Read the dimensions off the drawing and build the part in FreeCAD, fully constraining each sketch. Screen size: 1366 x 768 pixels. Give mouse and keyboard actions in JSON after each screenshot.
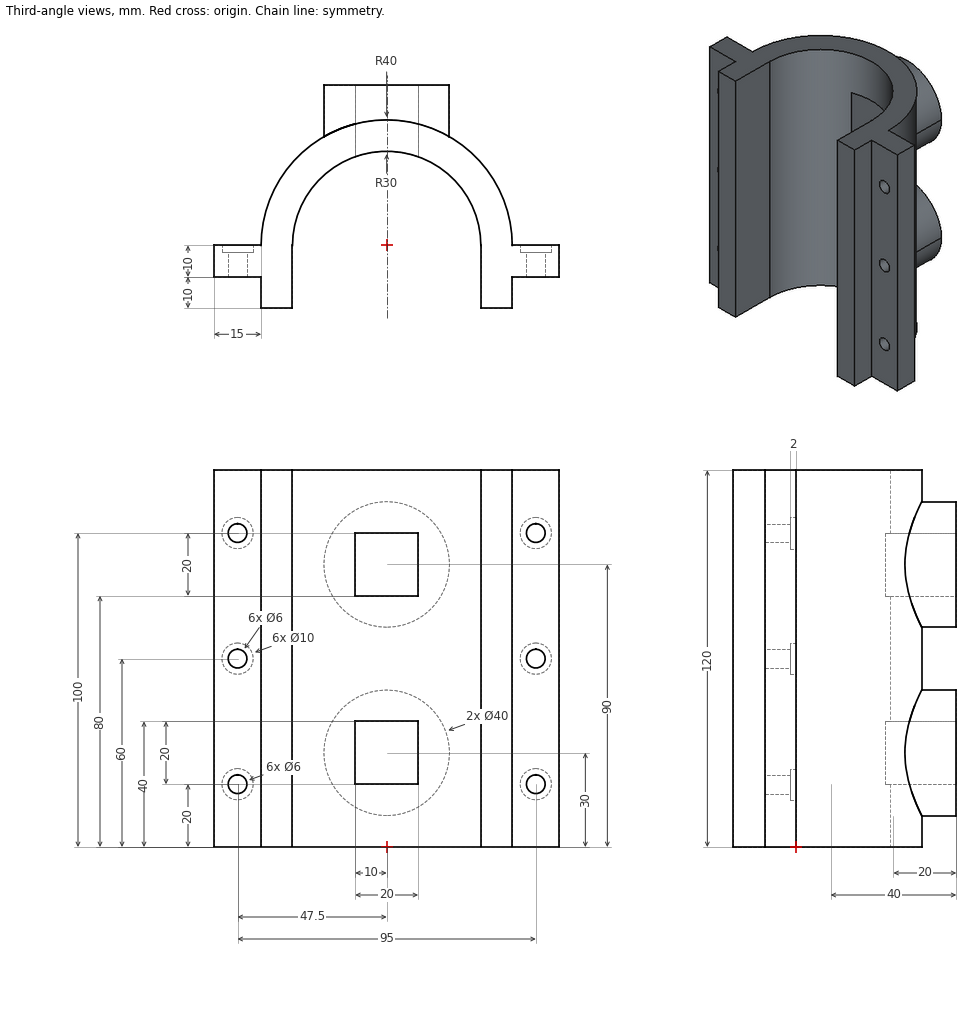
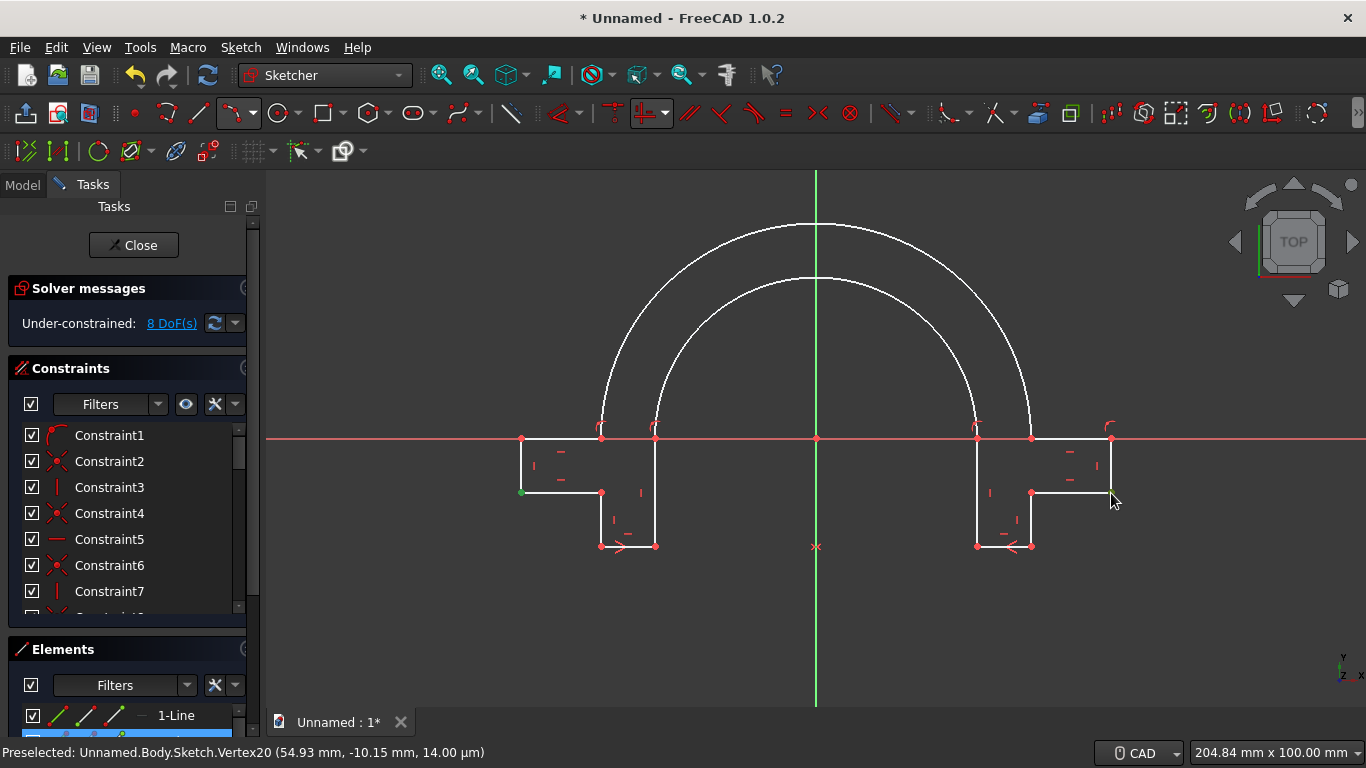
{"action": "left_click", "coordinate": [816, 645]}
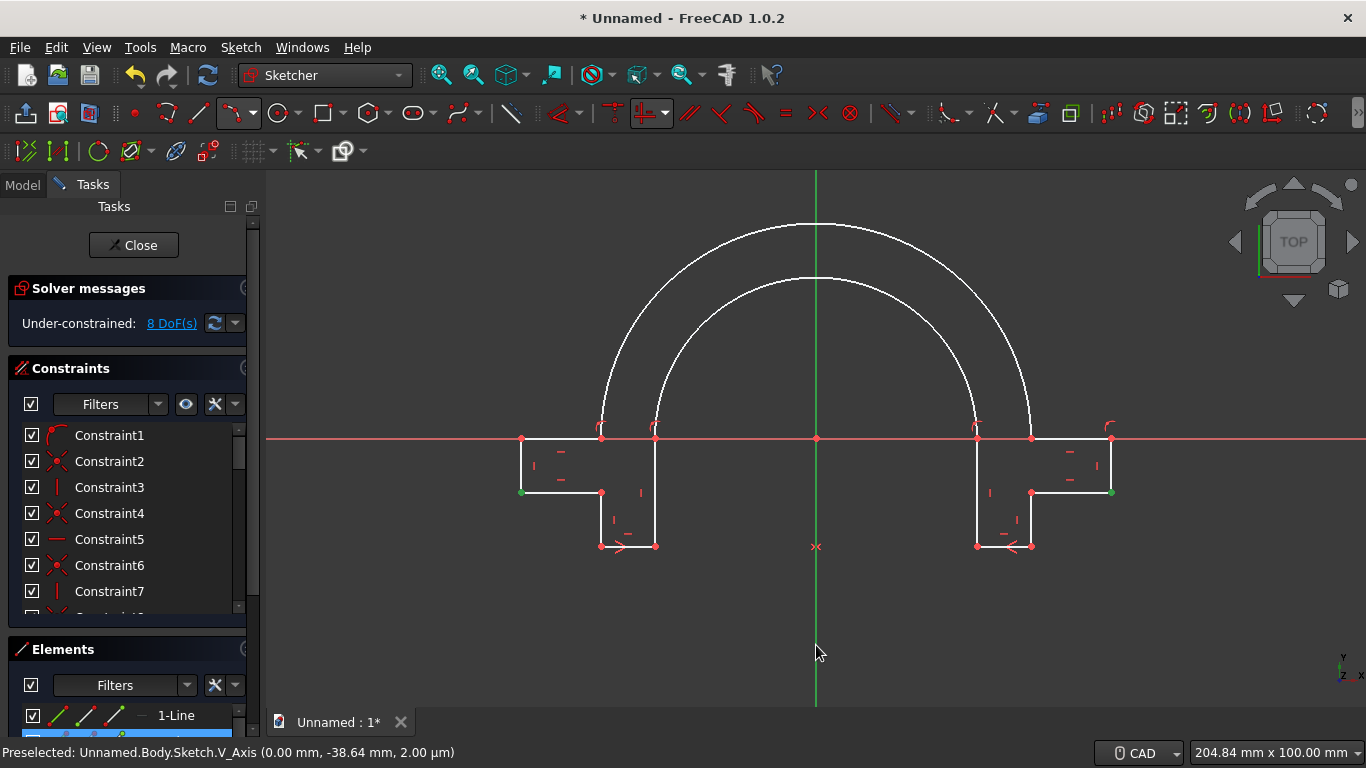
{"action": "left_click", "coordinate": [818, 114]}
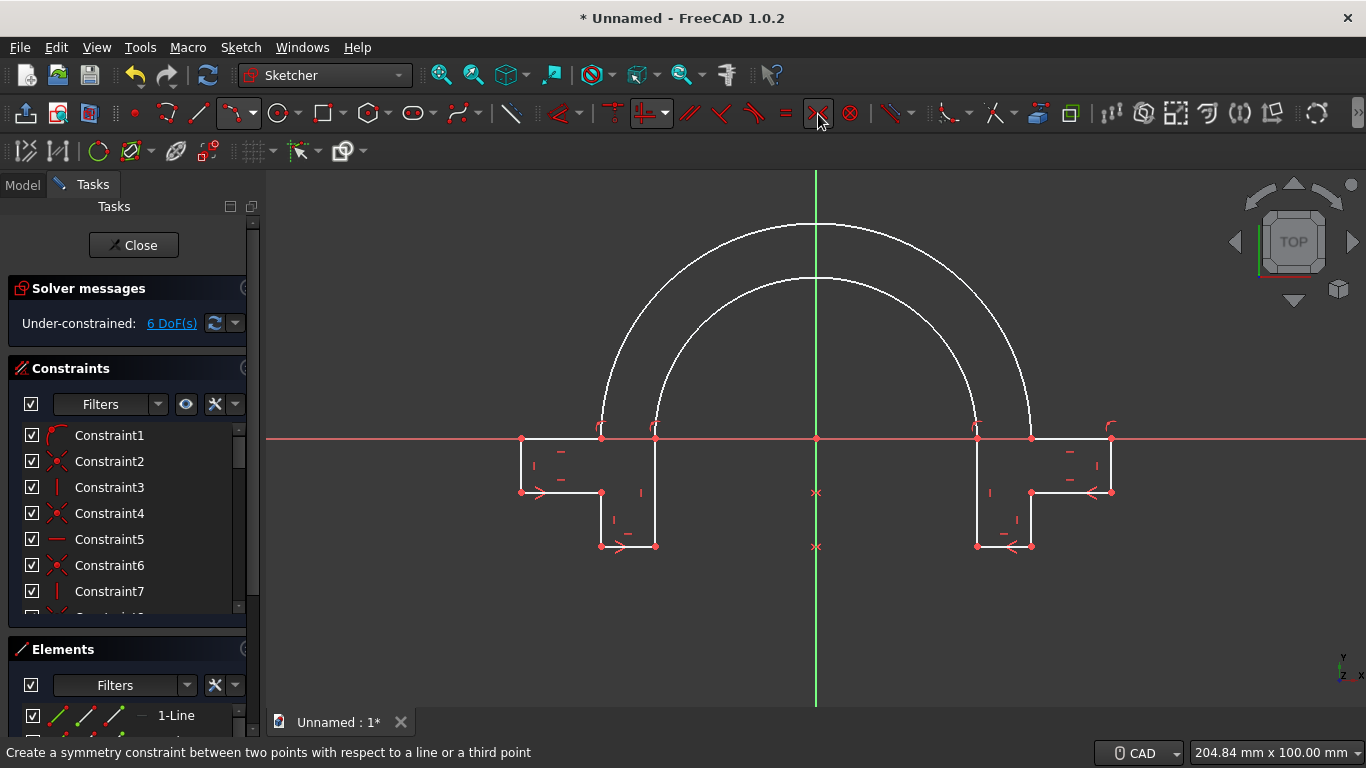
{"action": "left_click", "coordinate": [558, 114]}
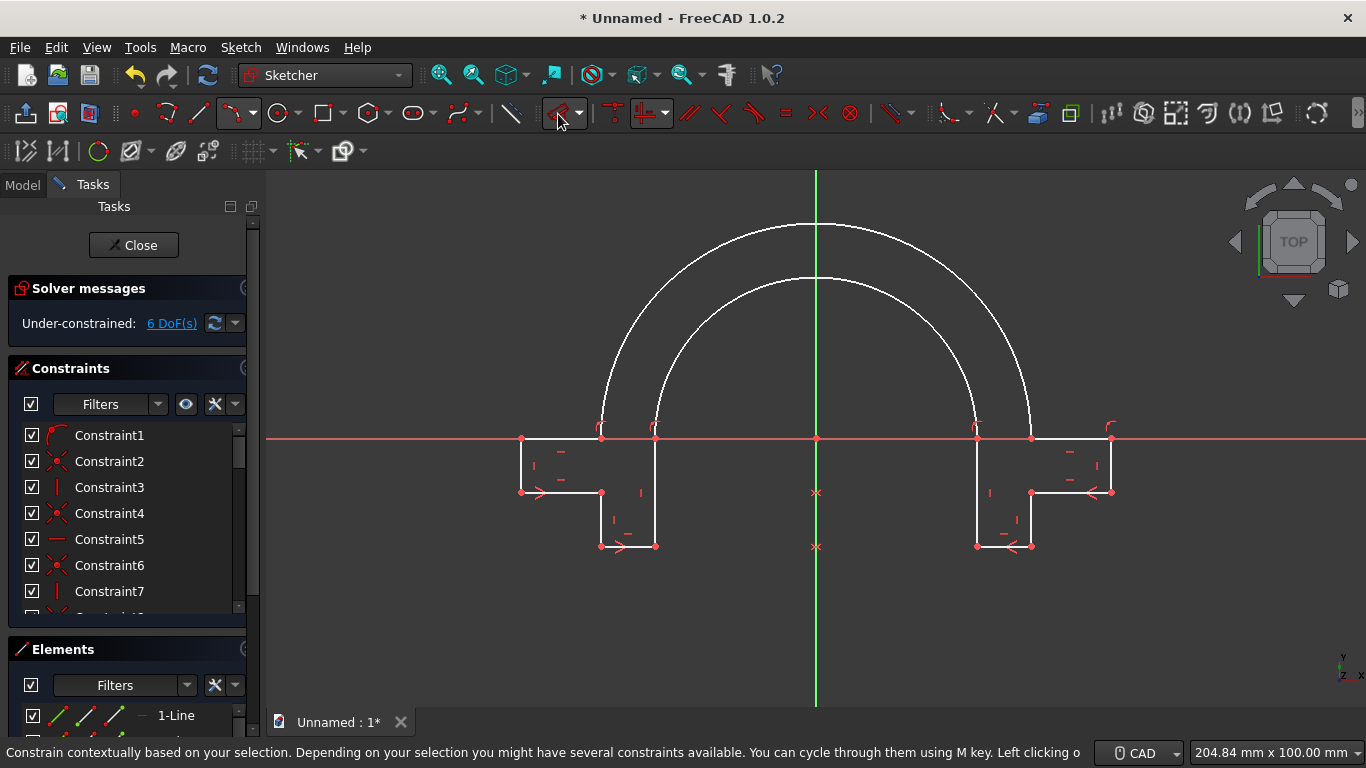
{"action": "left_click", "coordinate": [911, 308]}
{"action": "left_click", "coordinate": [930, 282]}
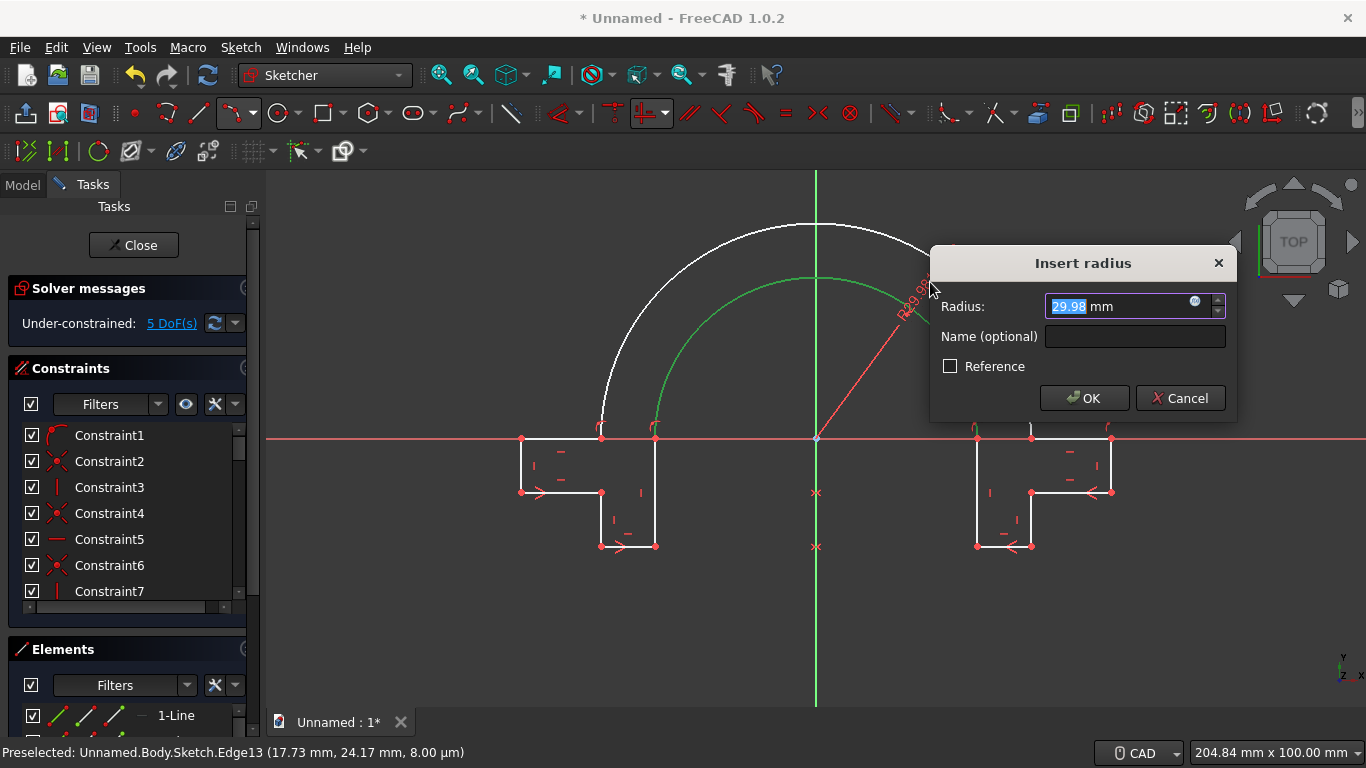
{"action": "type", "text": "30"}
{"action": "key", "text": "Return"}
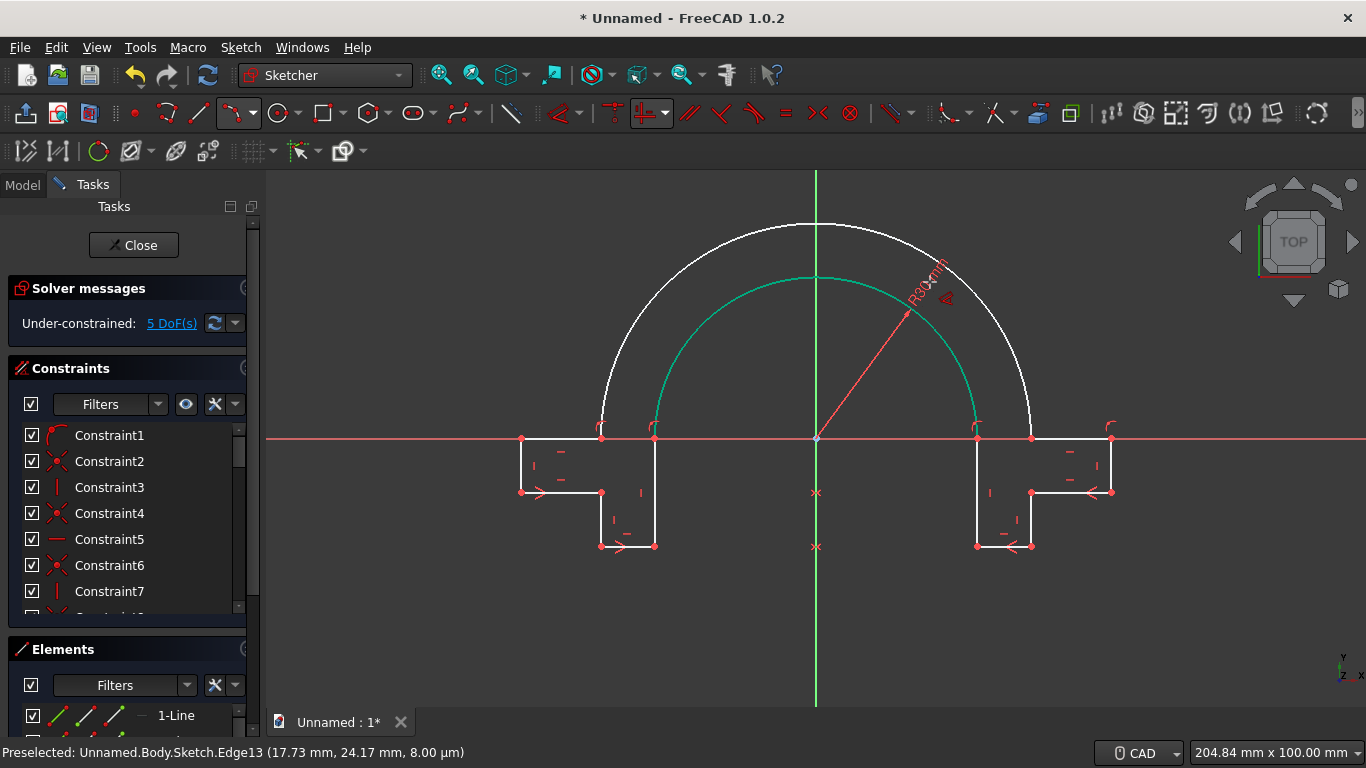
{"action": "left_click", "coordinate": [942, 265]}
{"action": "left_click", "coordinate": [961, 239]}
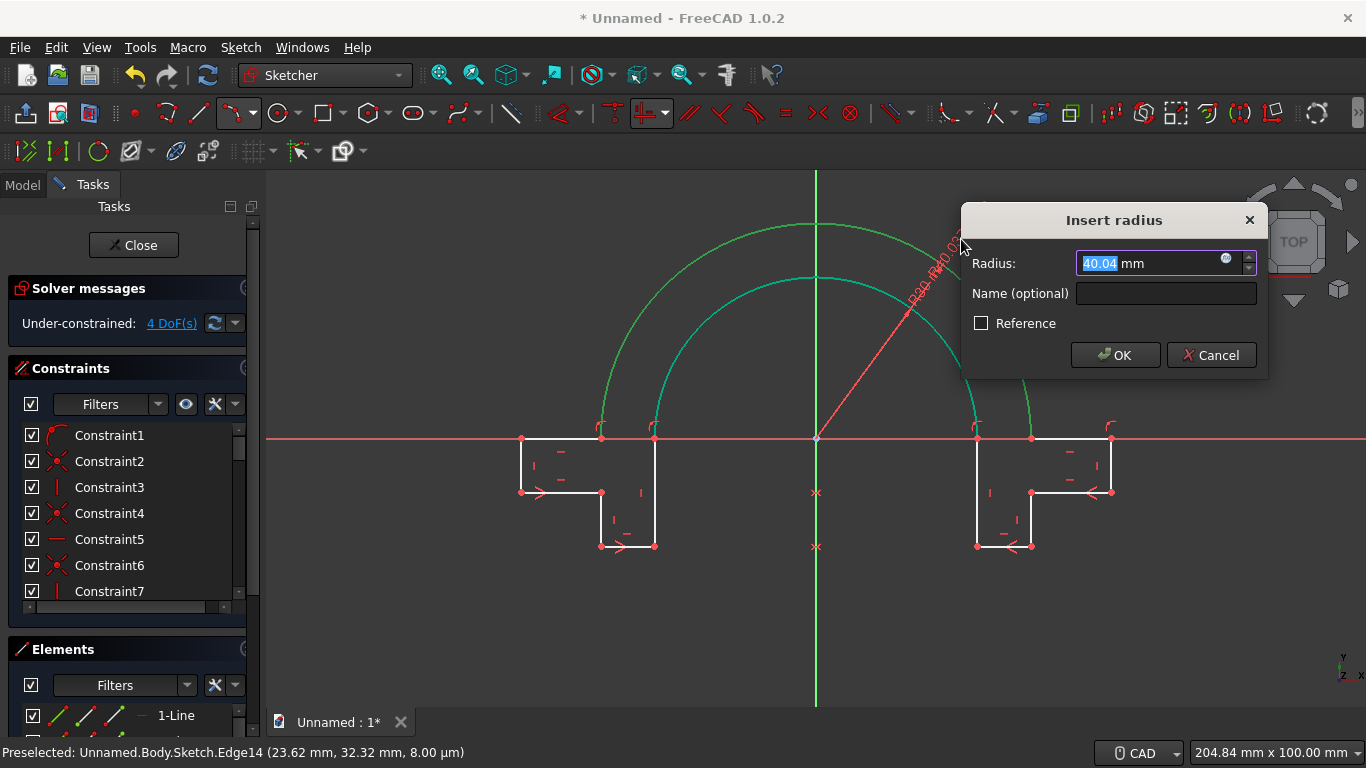
{"action": "type", "text": "40"}
{"action": "key", "text": "Return"}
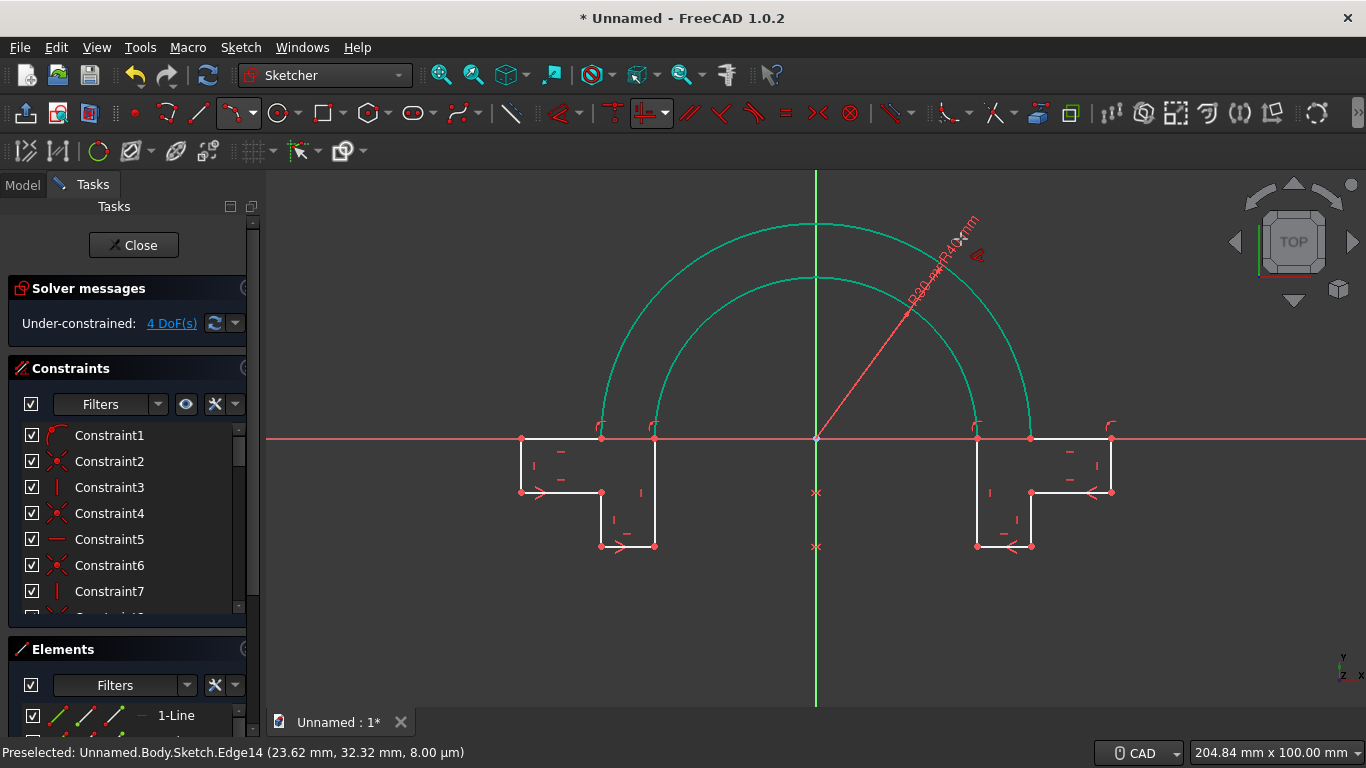
{"action": "left_click", "coordinate": [577, 438]}
{"action": "left_click", "coordinate": [561, 472]}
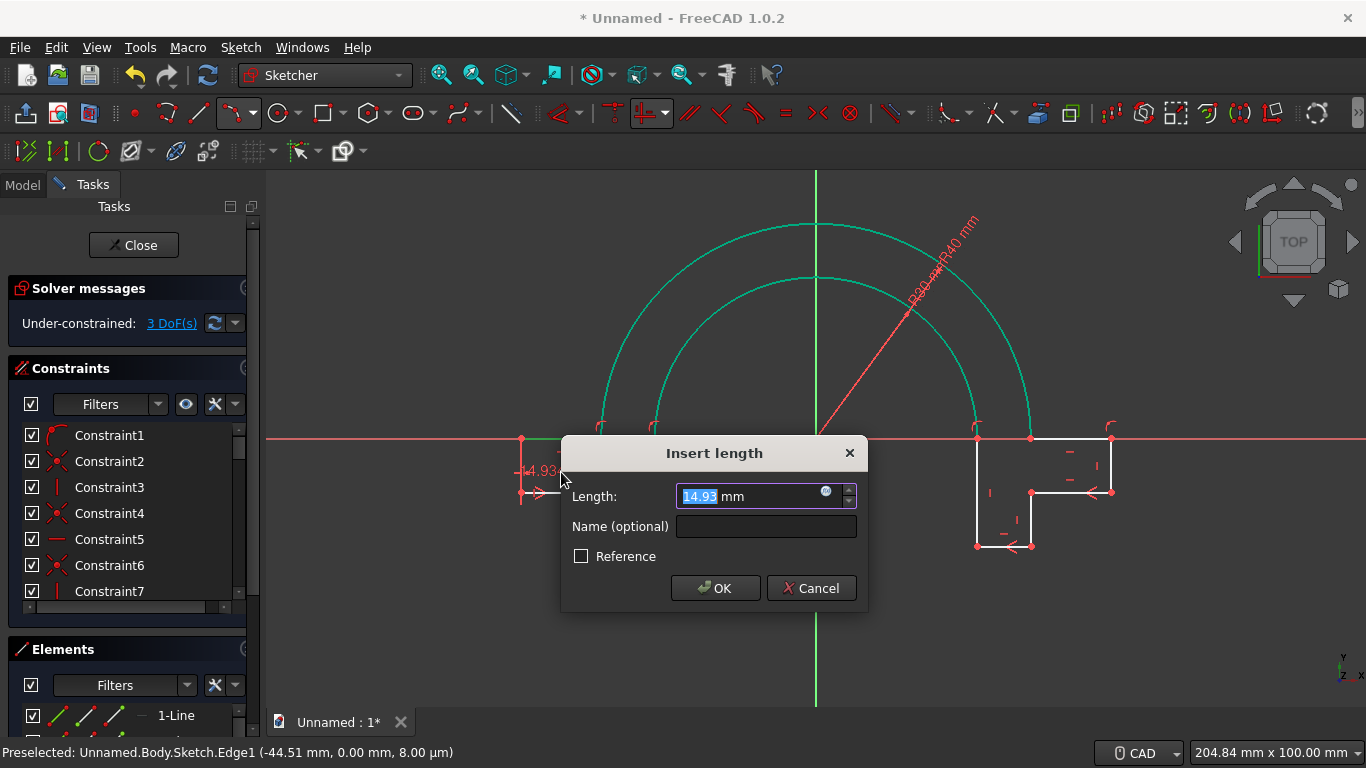
{"action": "type", "text": "15"}
{"action": "key", "text": "Return"}